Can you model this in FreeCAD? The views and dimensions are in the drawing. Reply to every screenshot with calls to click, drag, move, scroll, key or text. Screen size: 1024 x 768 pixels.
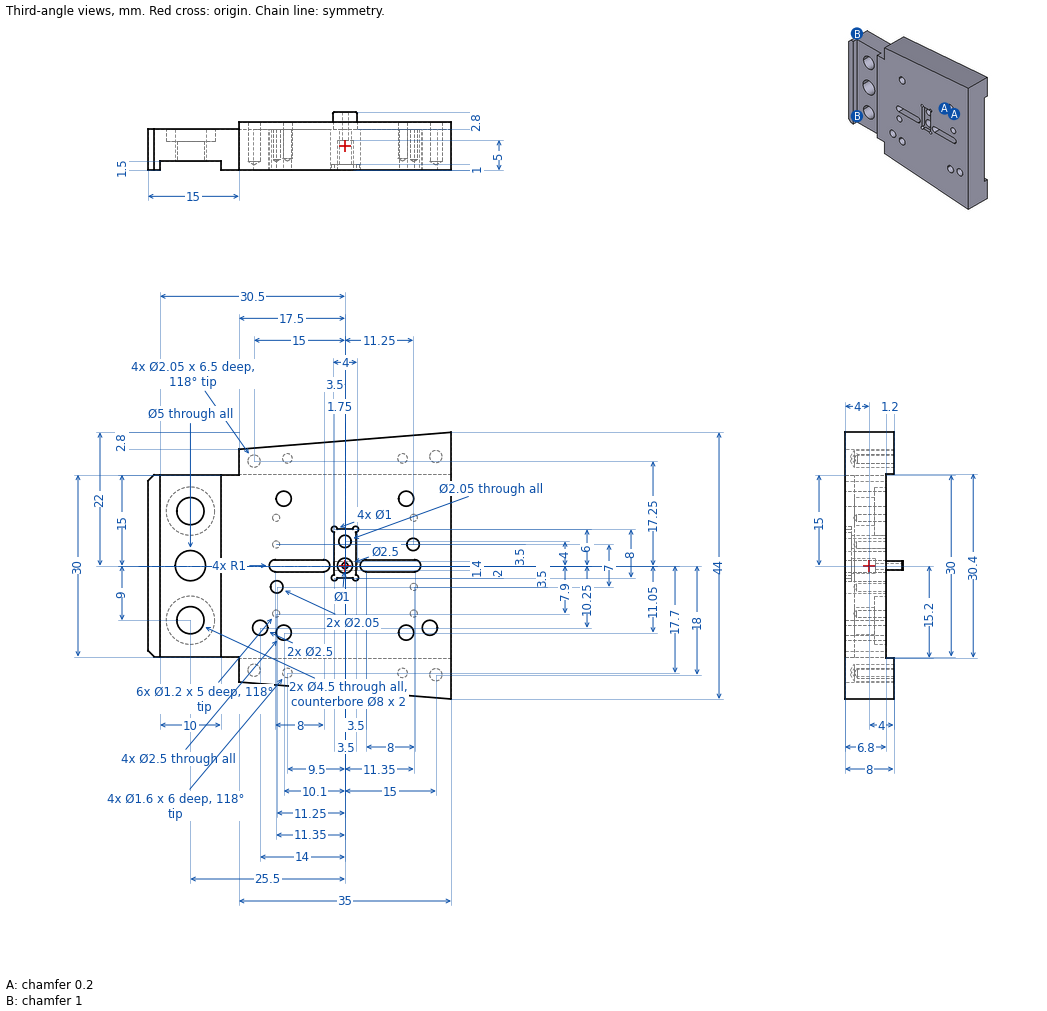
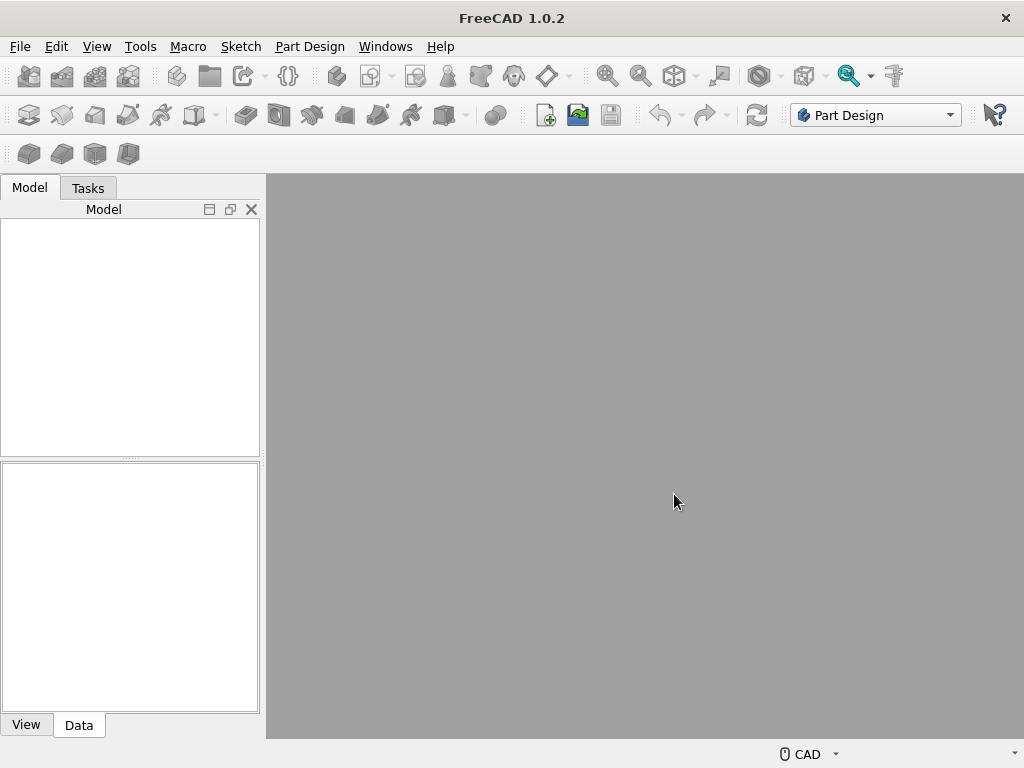
click(545, 116)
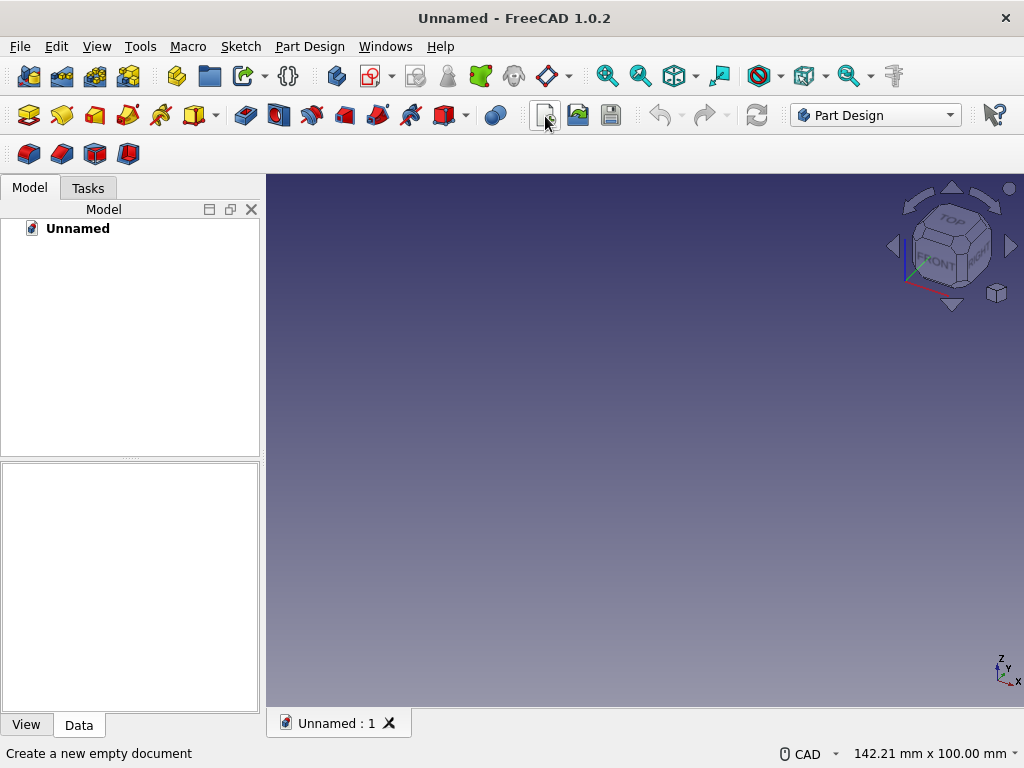
click(370, 76)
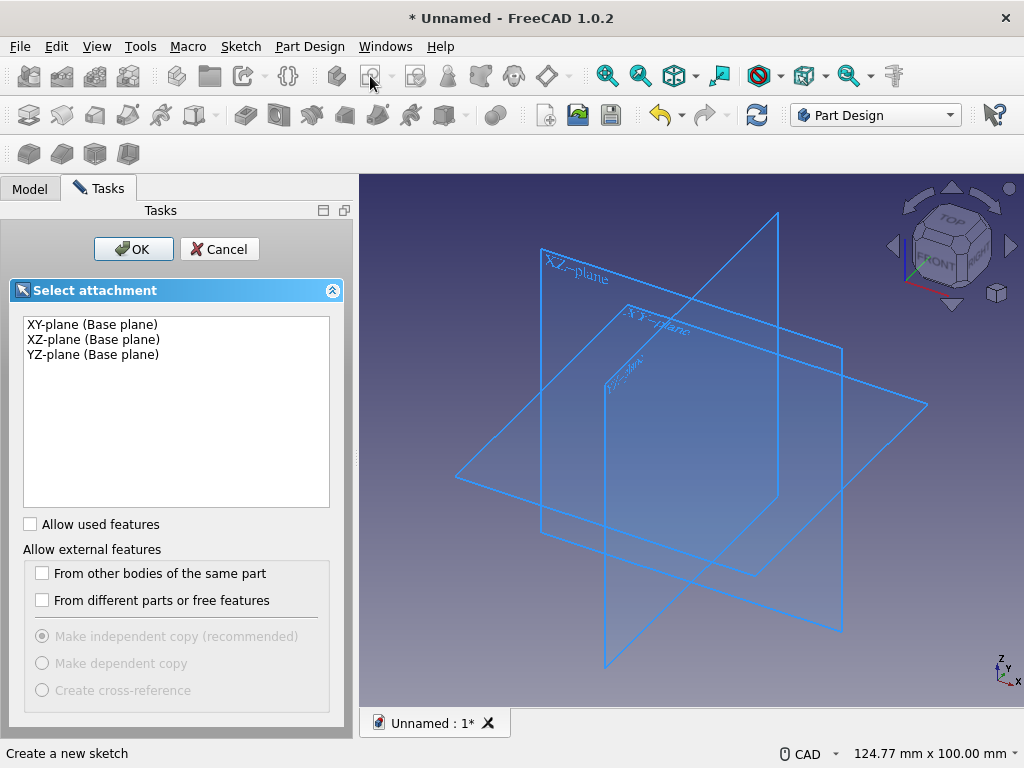
click(84, 340)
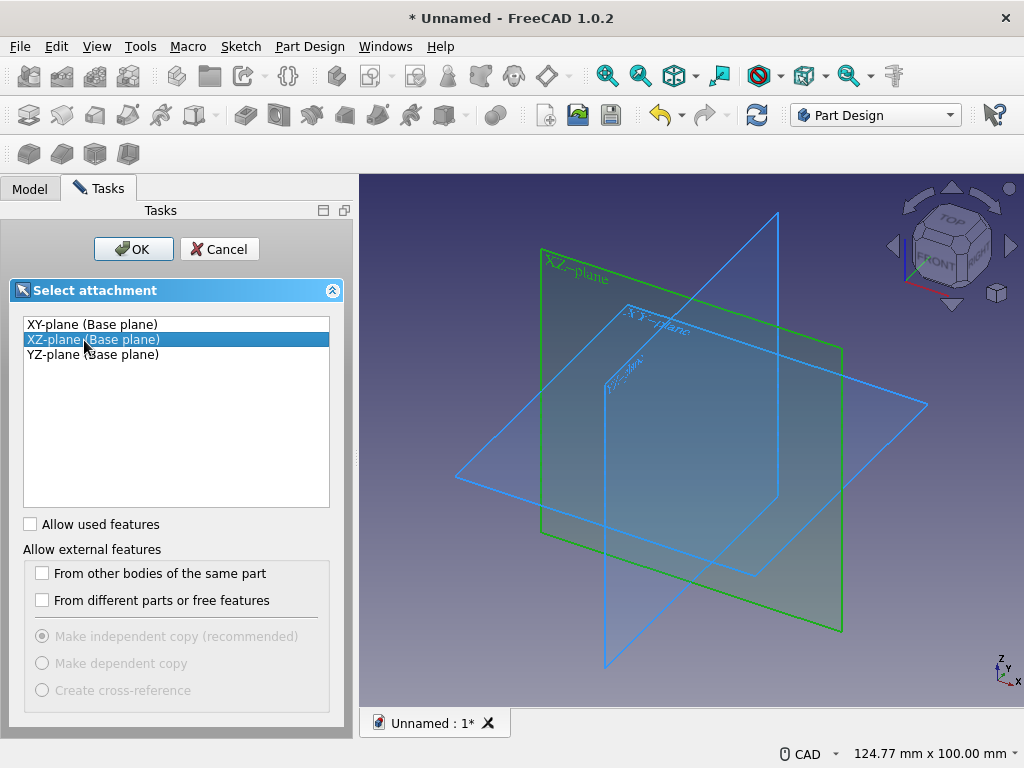
click(134, 249)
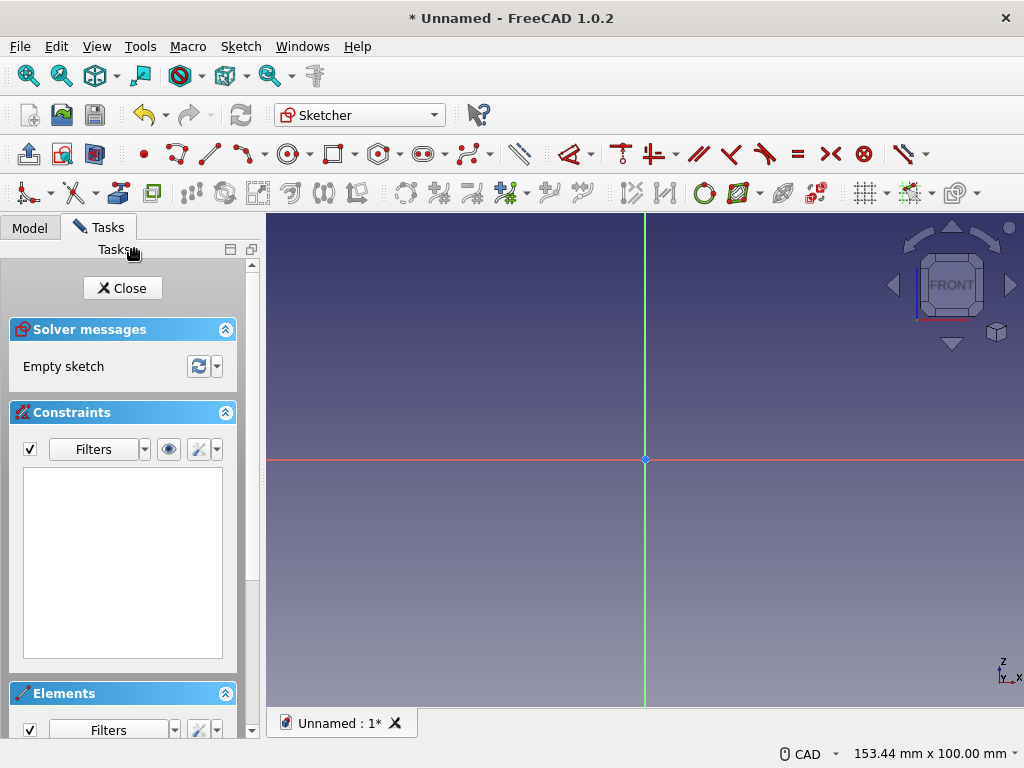
scroll(784, 460, up, 2)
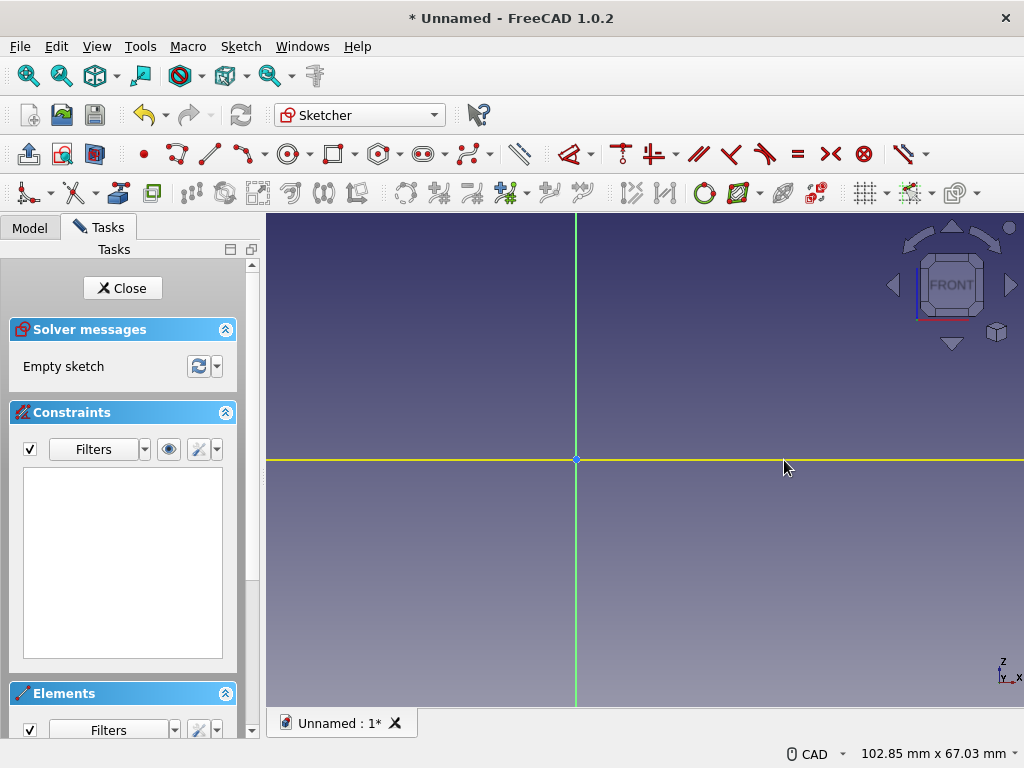
click(354, 154)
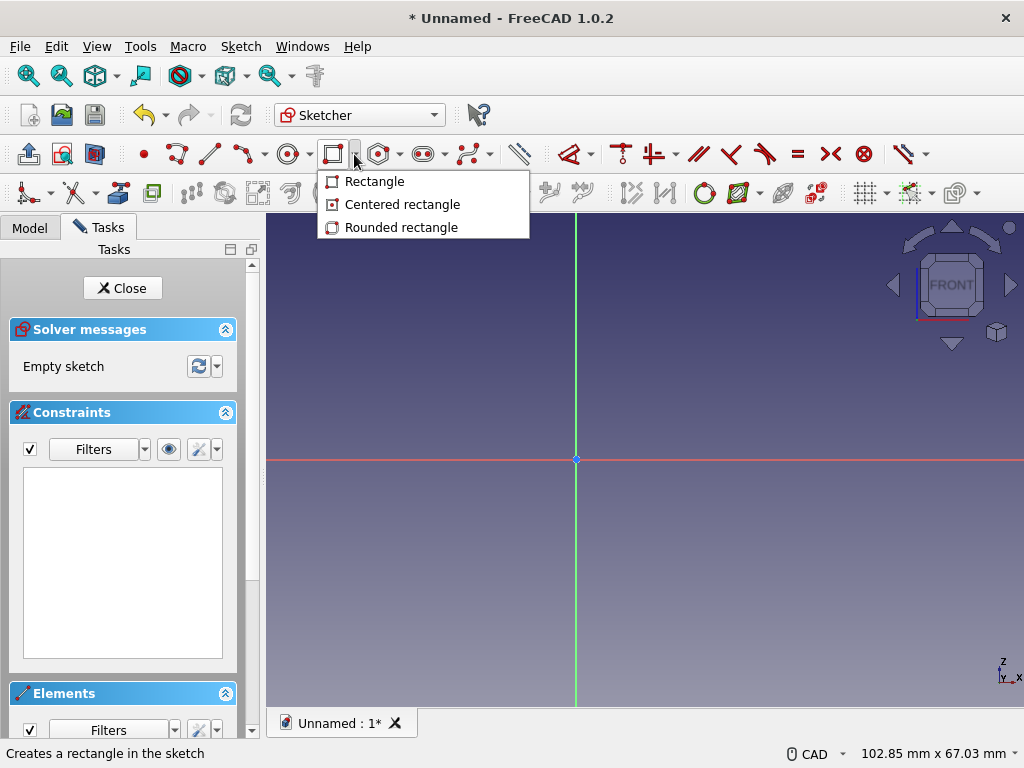
click(424, 204)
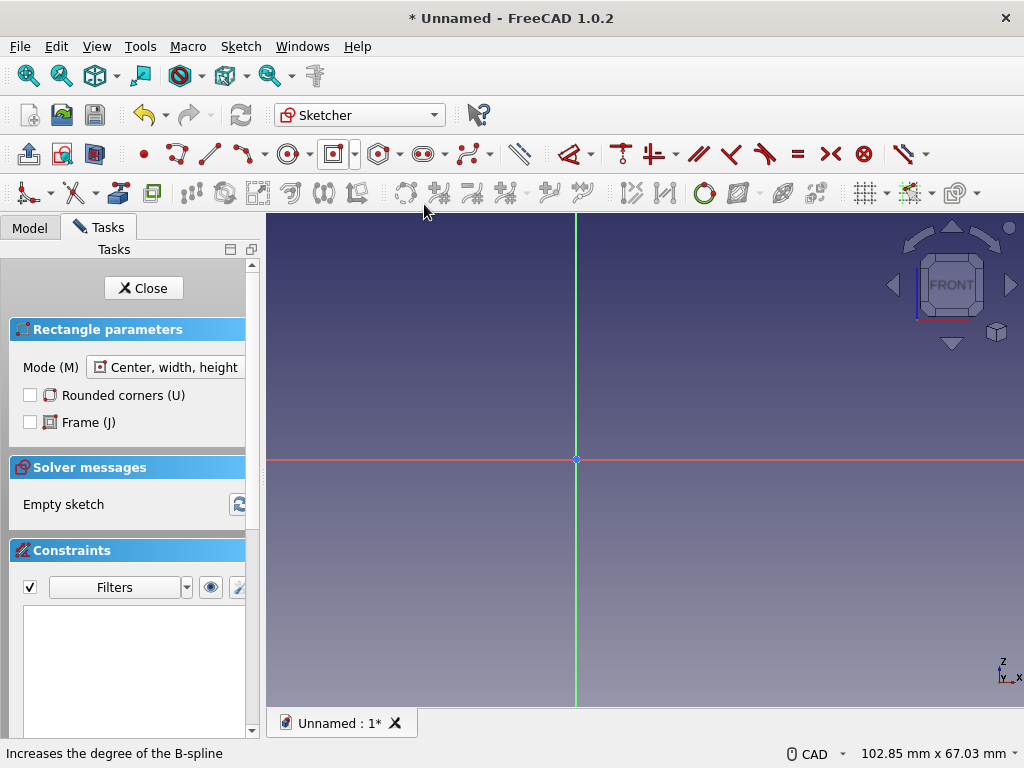
click(576, 460)
move(705, 298)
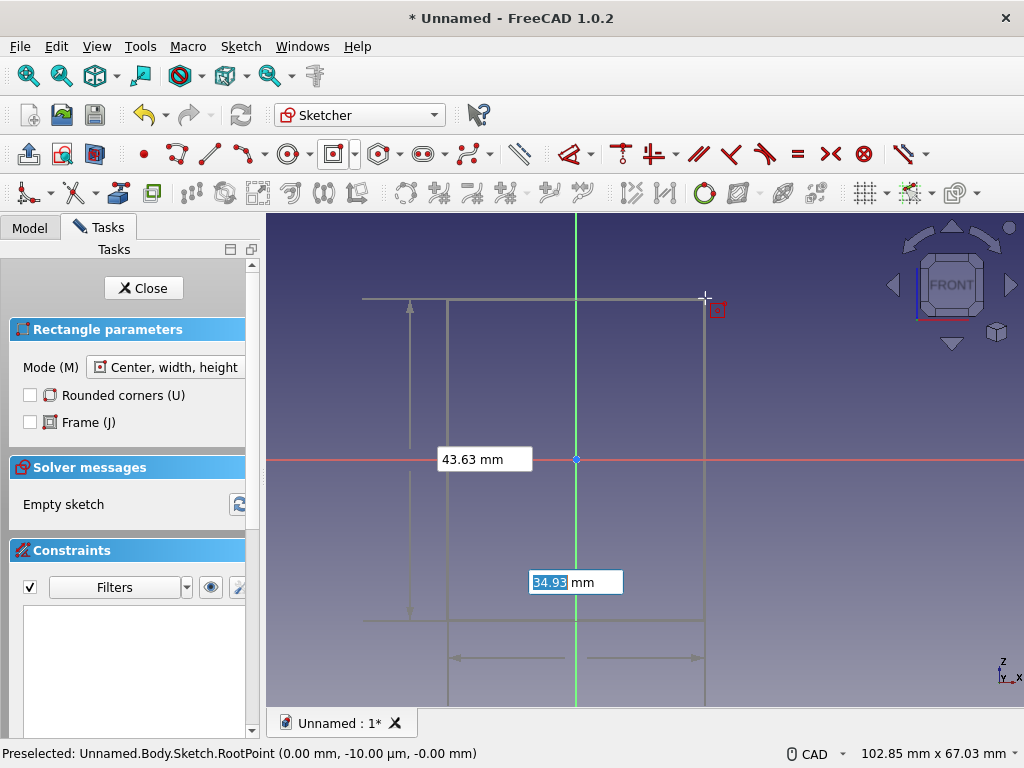
text(35)
key(Tab)
text(44)
key(Return)
key(Escape)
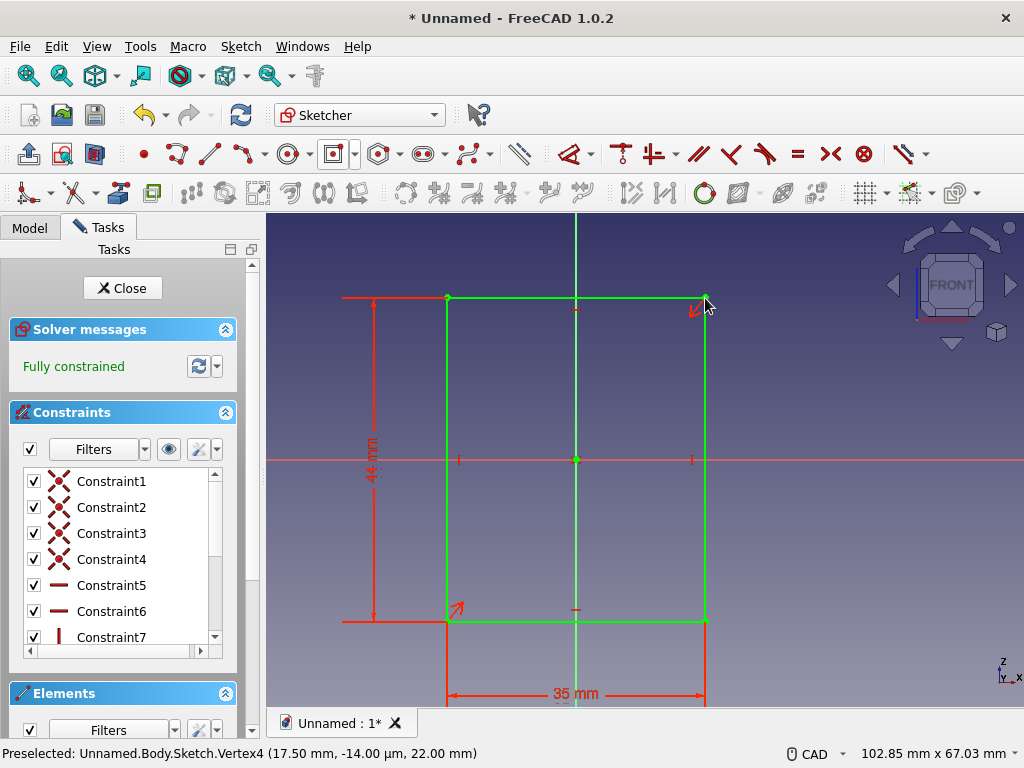
click(123, 288)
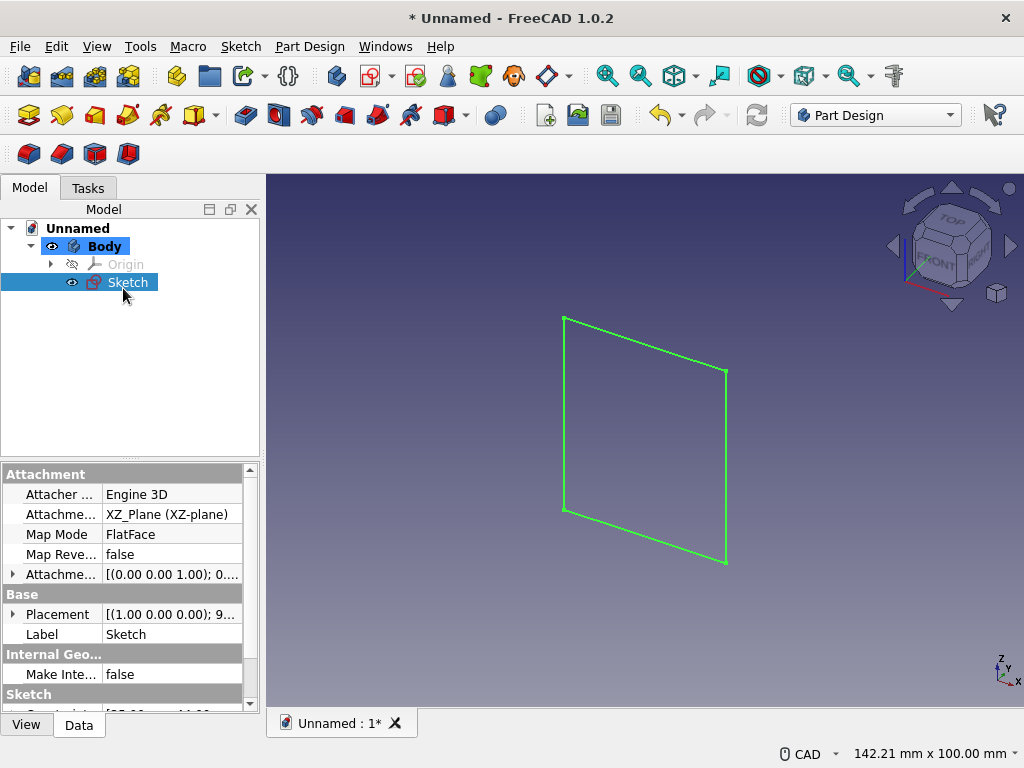
click(29, 116)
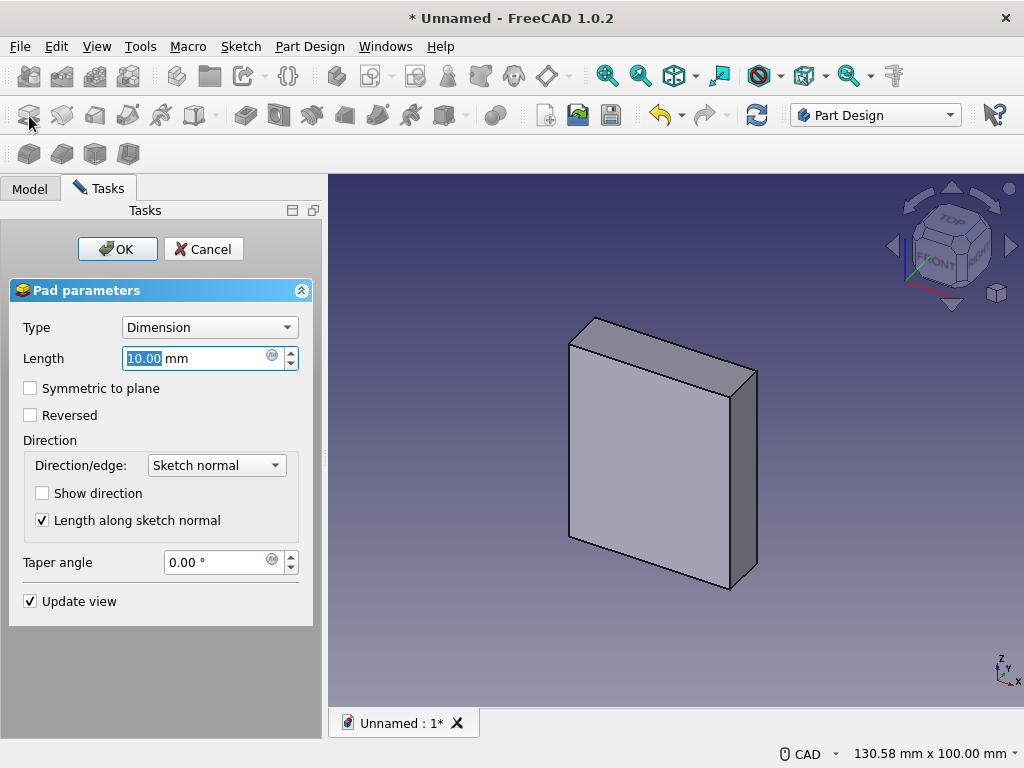
text(8)
key(Tab)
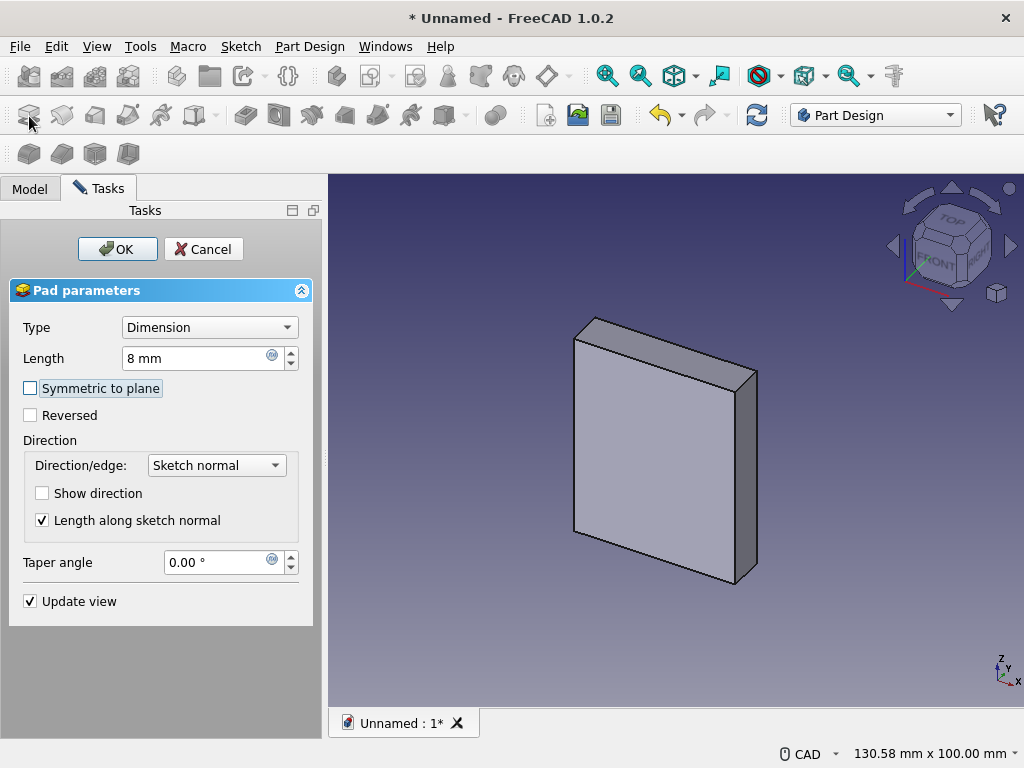
click(31, 388)